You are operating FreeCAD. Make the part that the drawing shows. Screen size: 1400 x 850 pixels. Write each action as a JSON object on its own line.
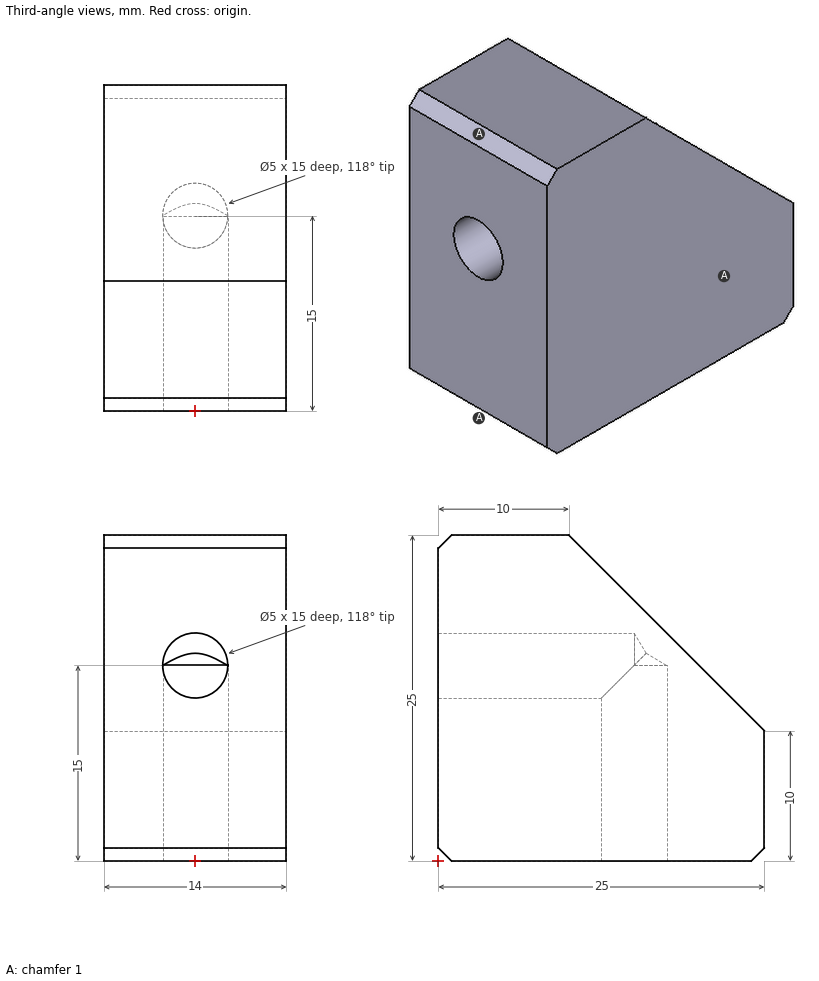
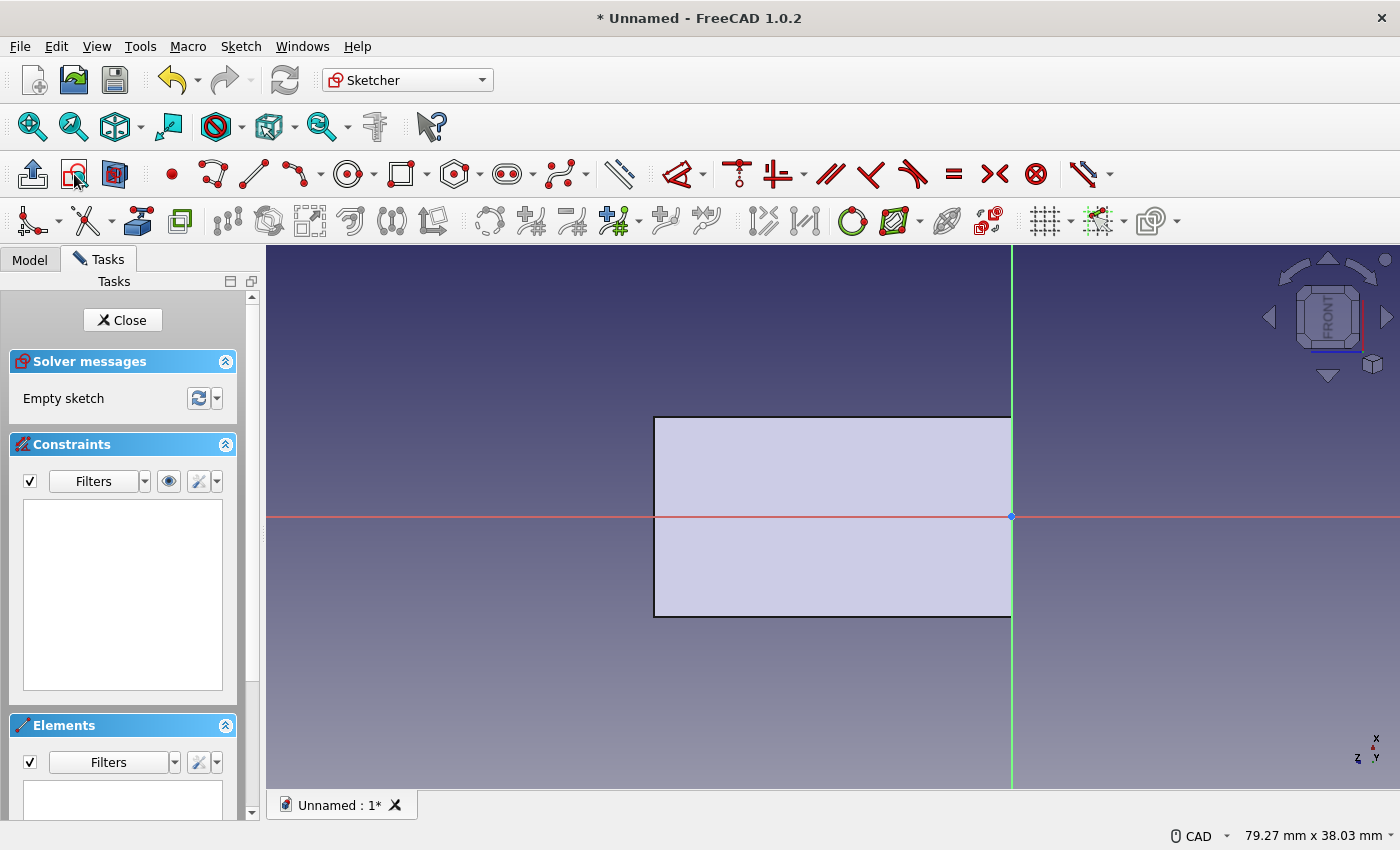
{"action": "scroll", "coordinate": [806, 517], "scroll_direction": "up", "scroll_amount": 8}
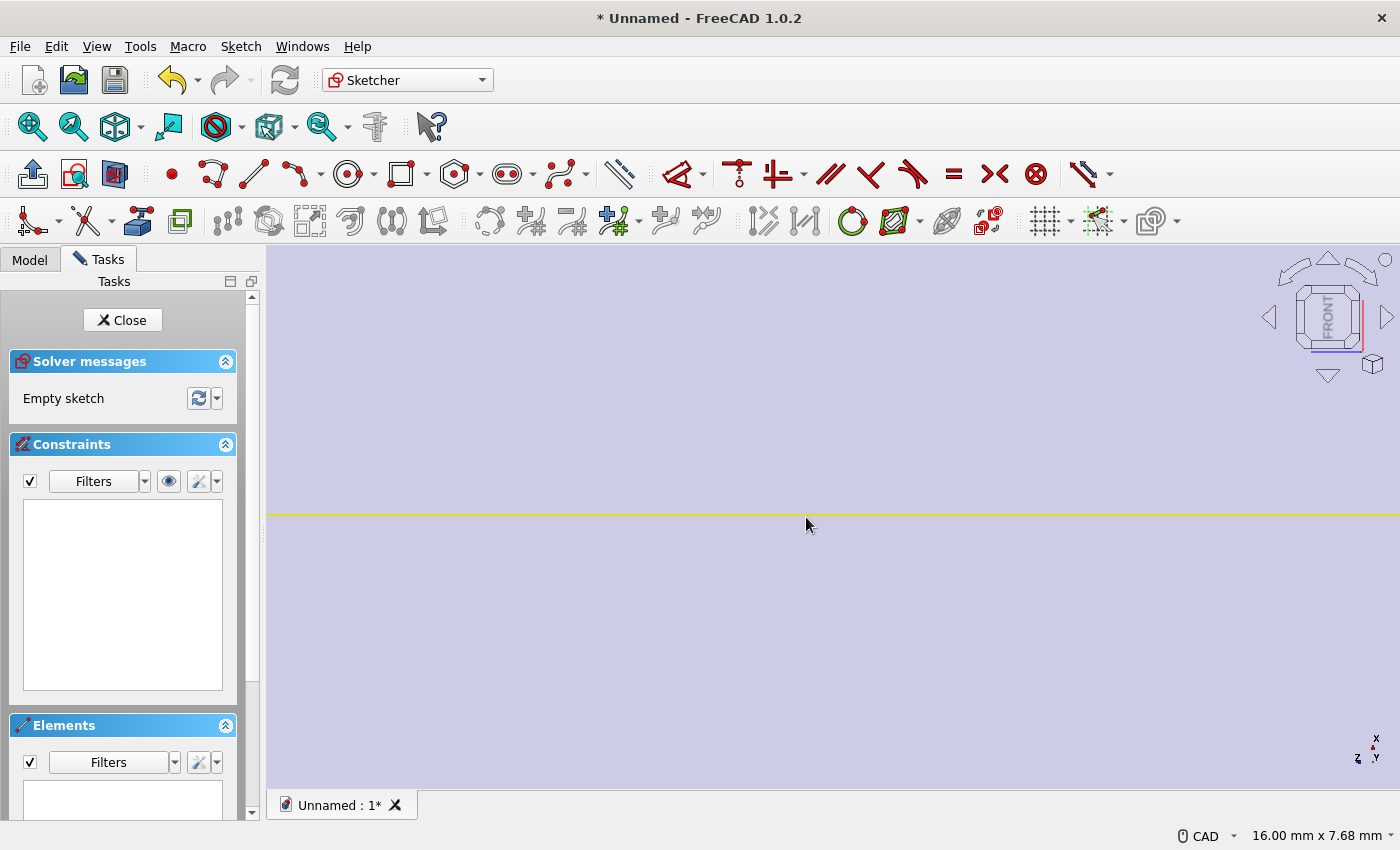
{"action": "left_click", "coordinate": [348, 174]}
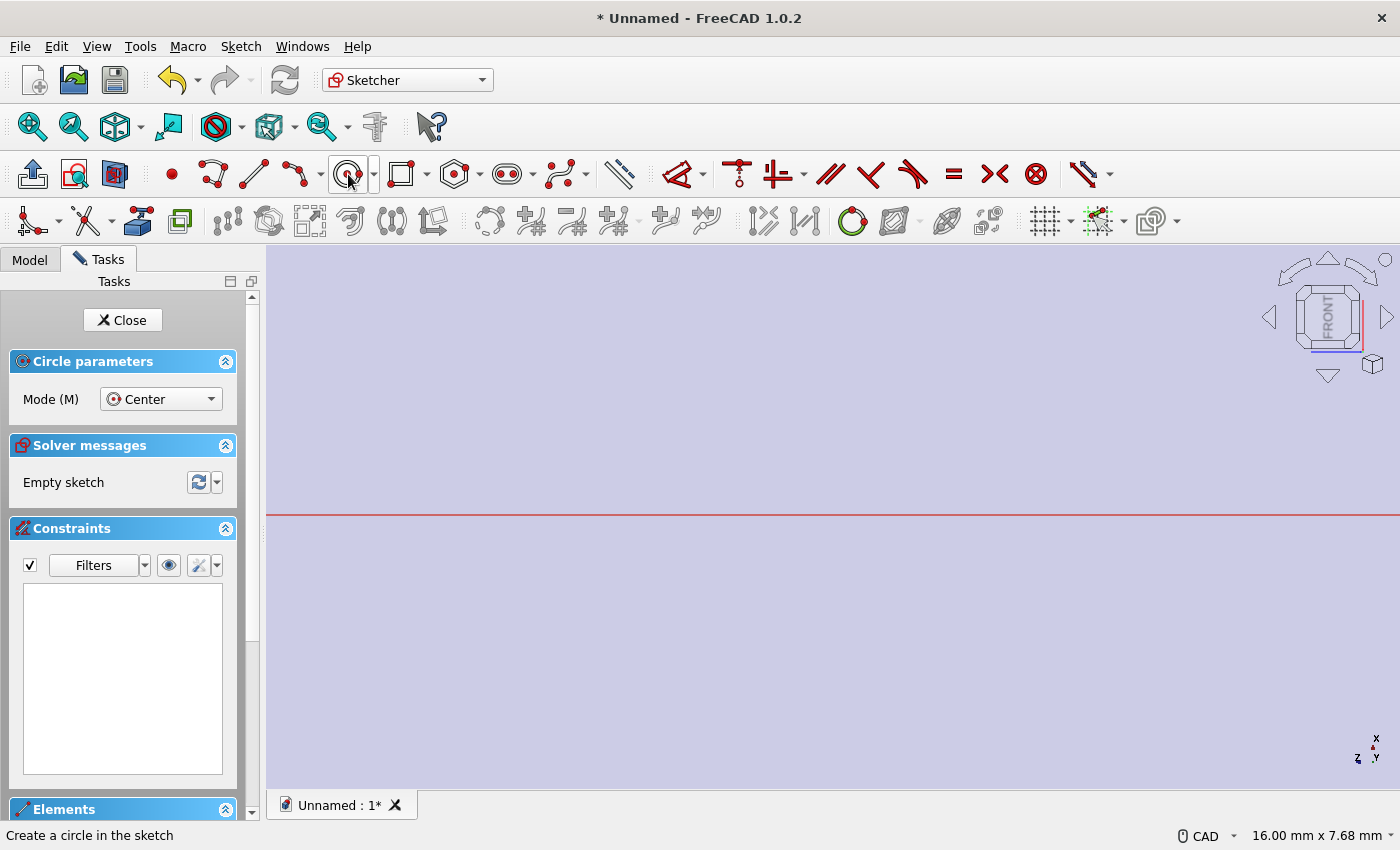
{"action": "left_click", "coordinate": [761, 515]}
{"action": "left_click", "coordinate": [886, 390]}
{"action": "key", "text": "Escape"}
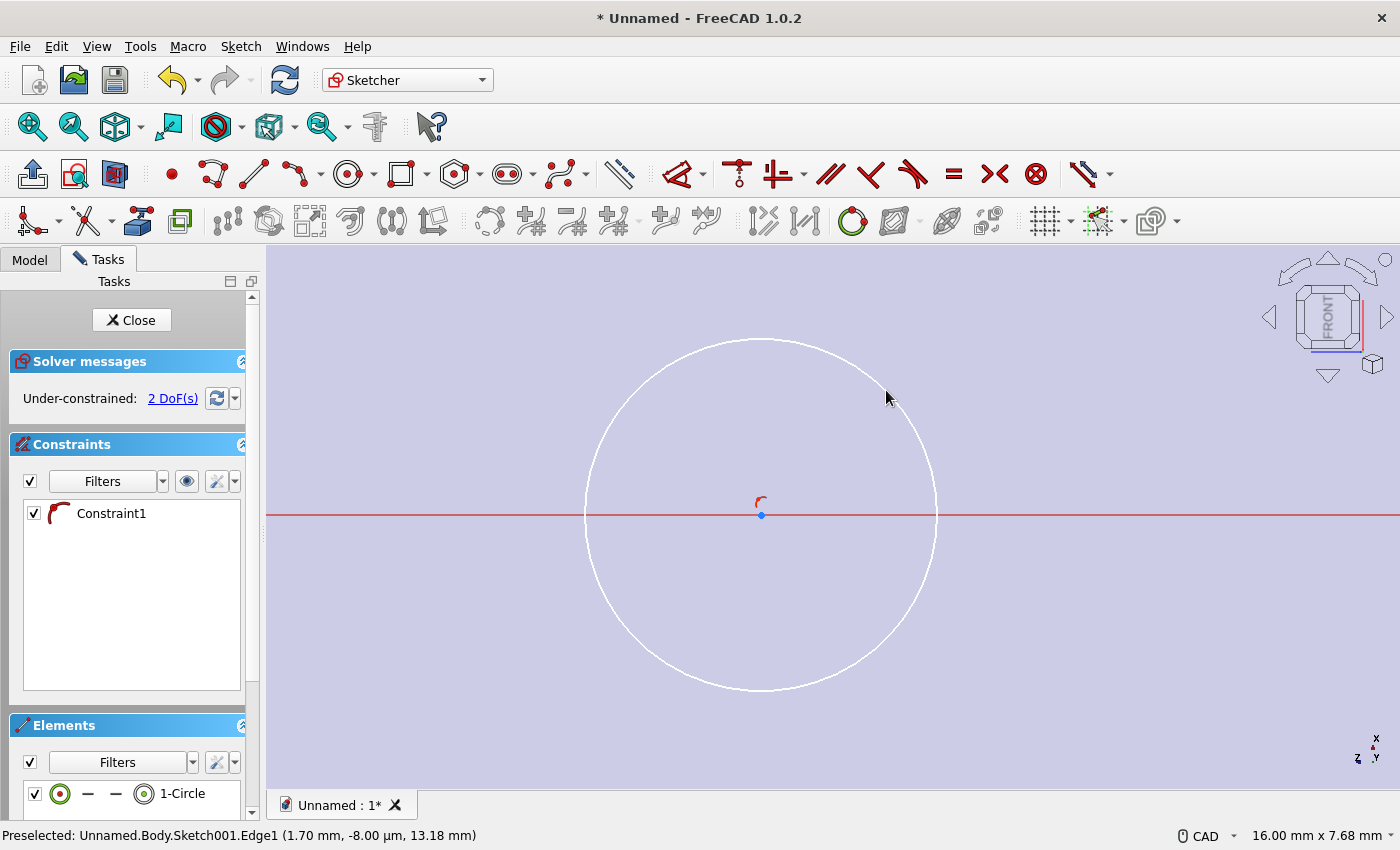
{"action": "left_click", "coordinate": [676, 174]}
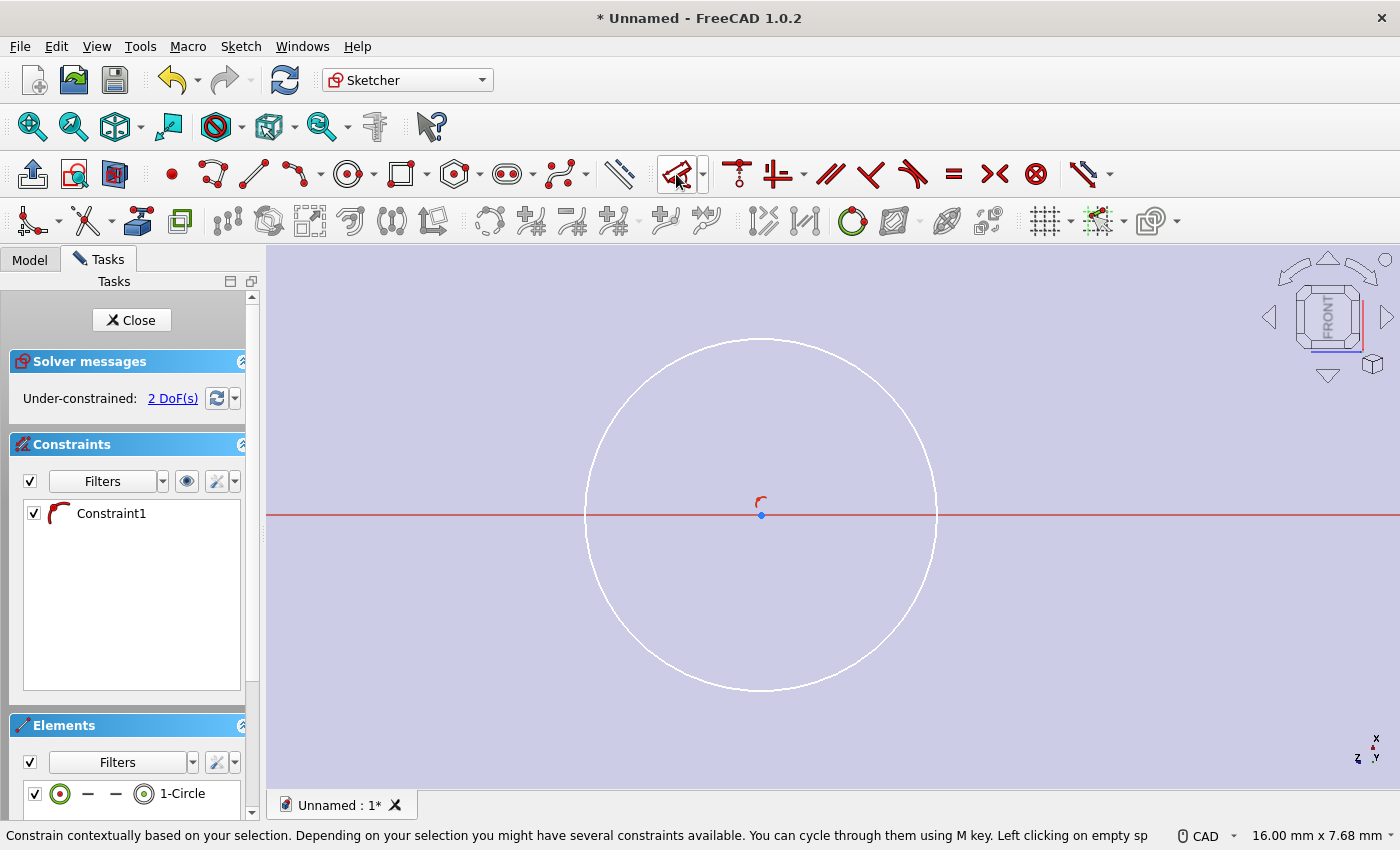
{"action": "left_click", "coordinate": [885, 390]}
{"action": "left_click", "coordinate": [908, 367]}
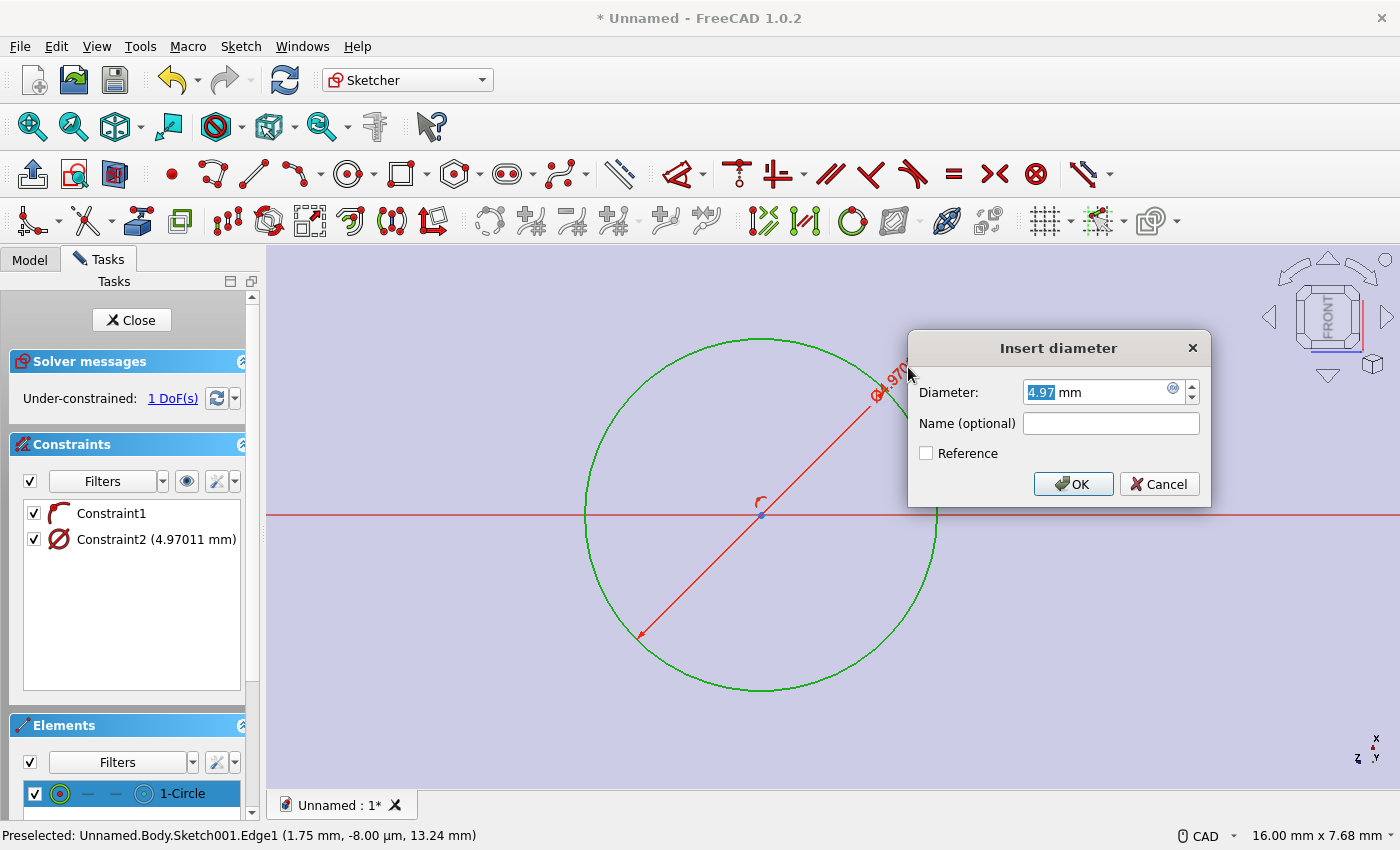
{"action": "type", "text": "5"}
{"action": "key", "text": "Return"}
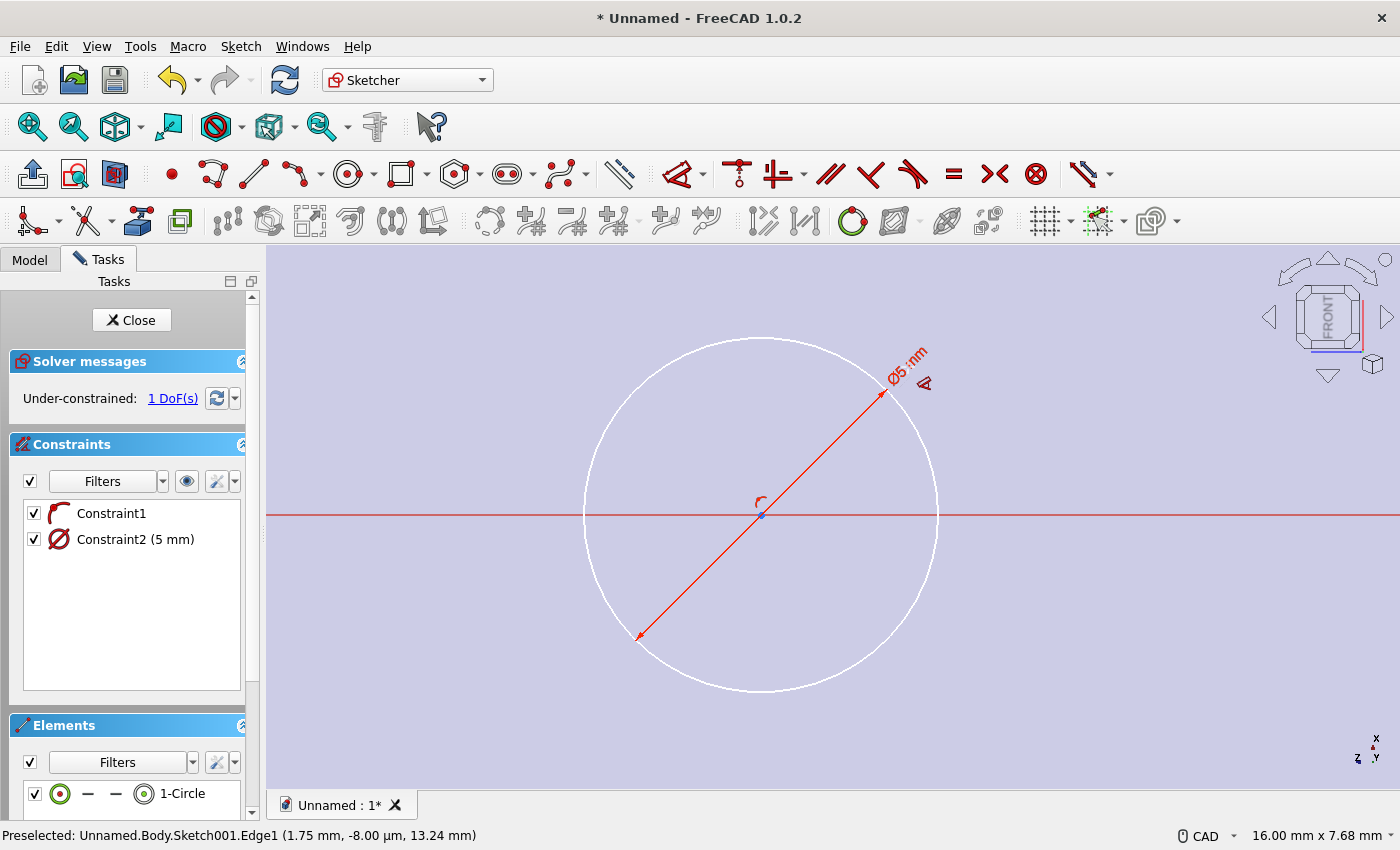
{"action": "left_click", "coordinate": [761, 515]}
{"action": "left_click", "coordinate": [998, 549]}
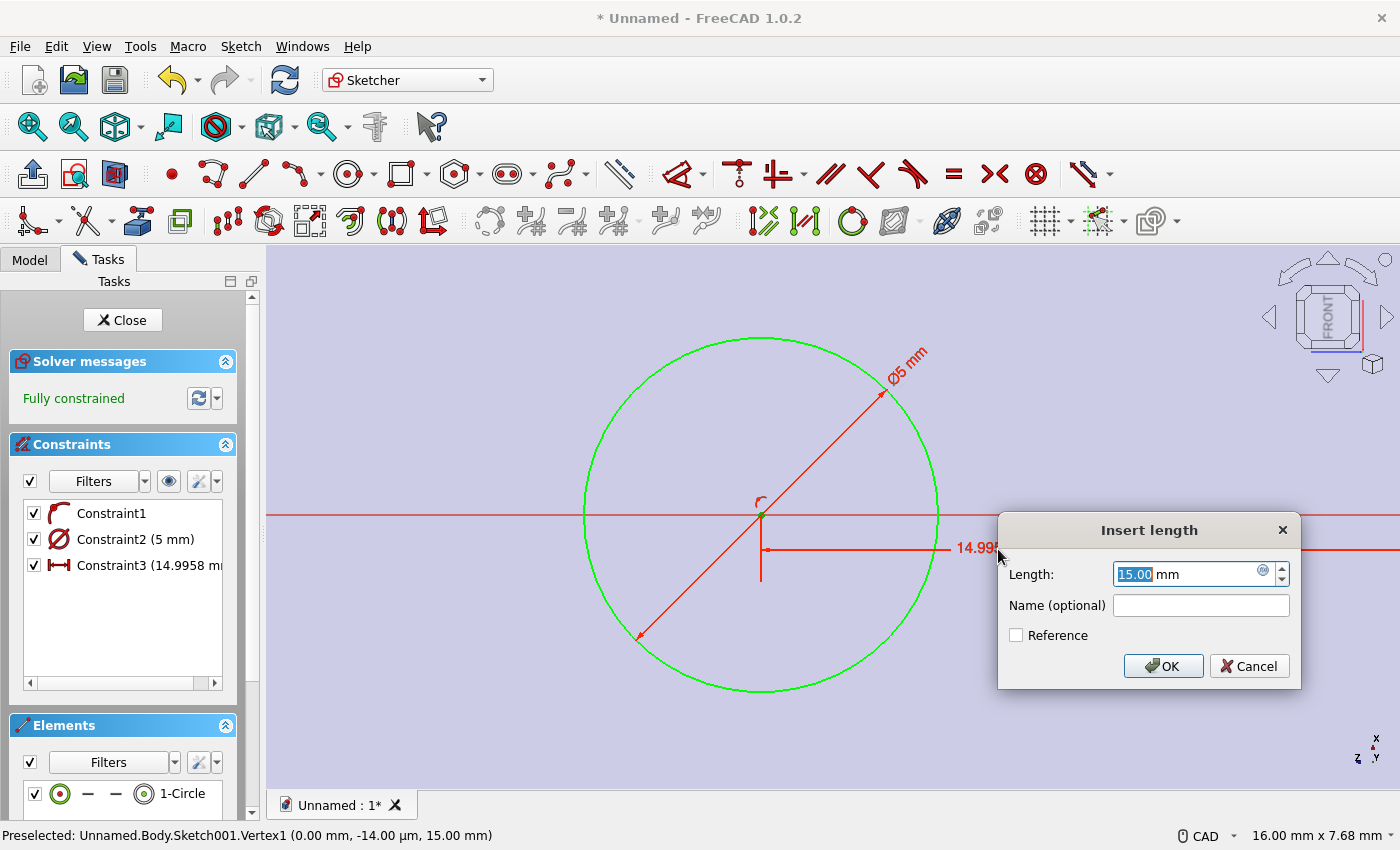
{"action": "type", "text": "15"}
{"action": "key", "text": "Return"}
{"action": "key", "text": "Escape"}